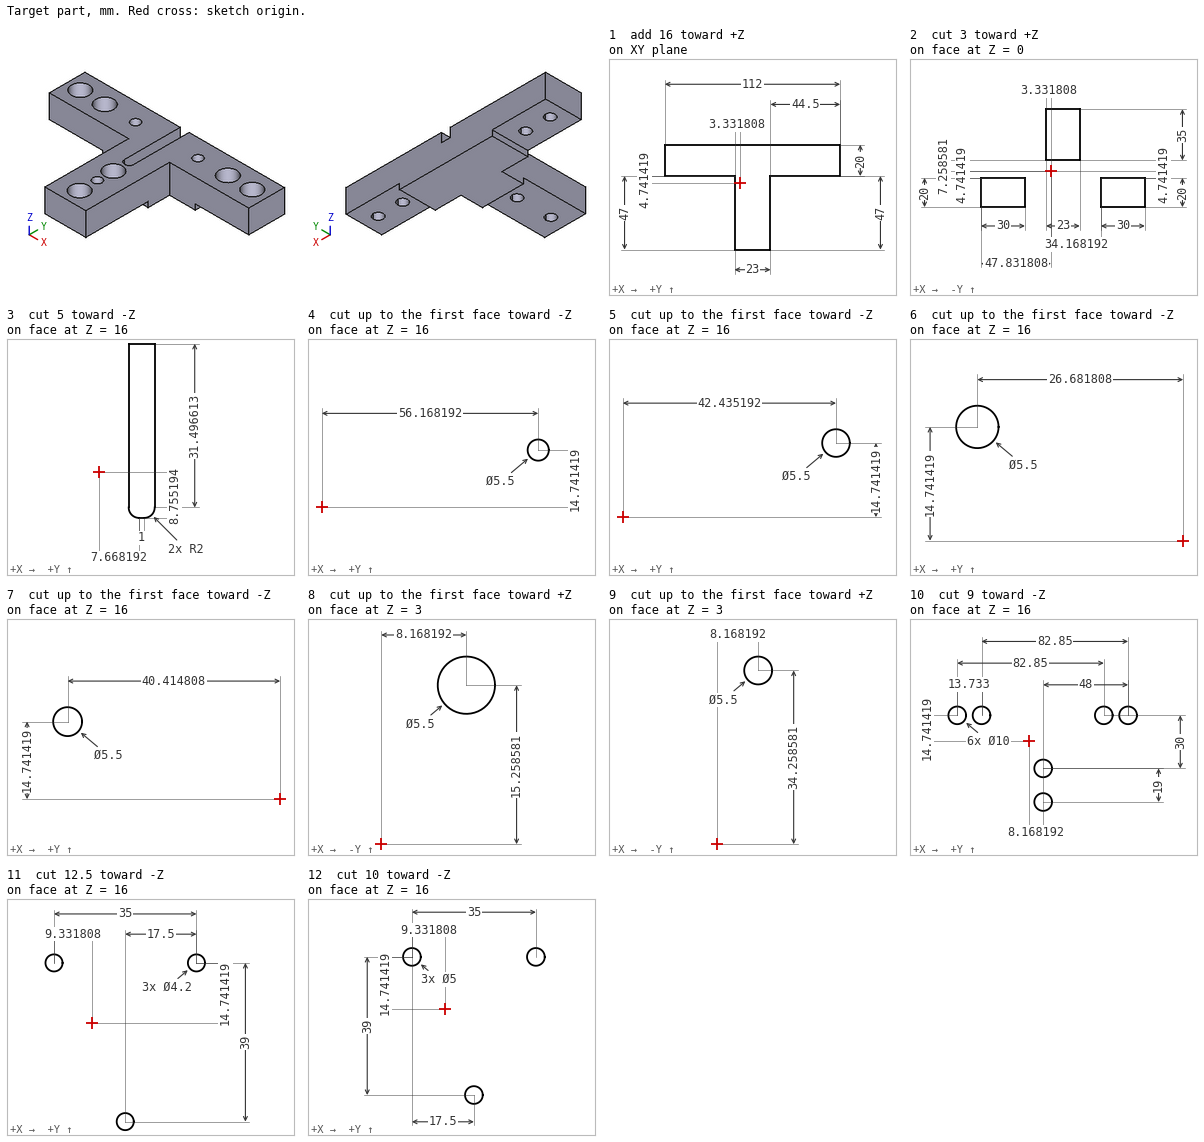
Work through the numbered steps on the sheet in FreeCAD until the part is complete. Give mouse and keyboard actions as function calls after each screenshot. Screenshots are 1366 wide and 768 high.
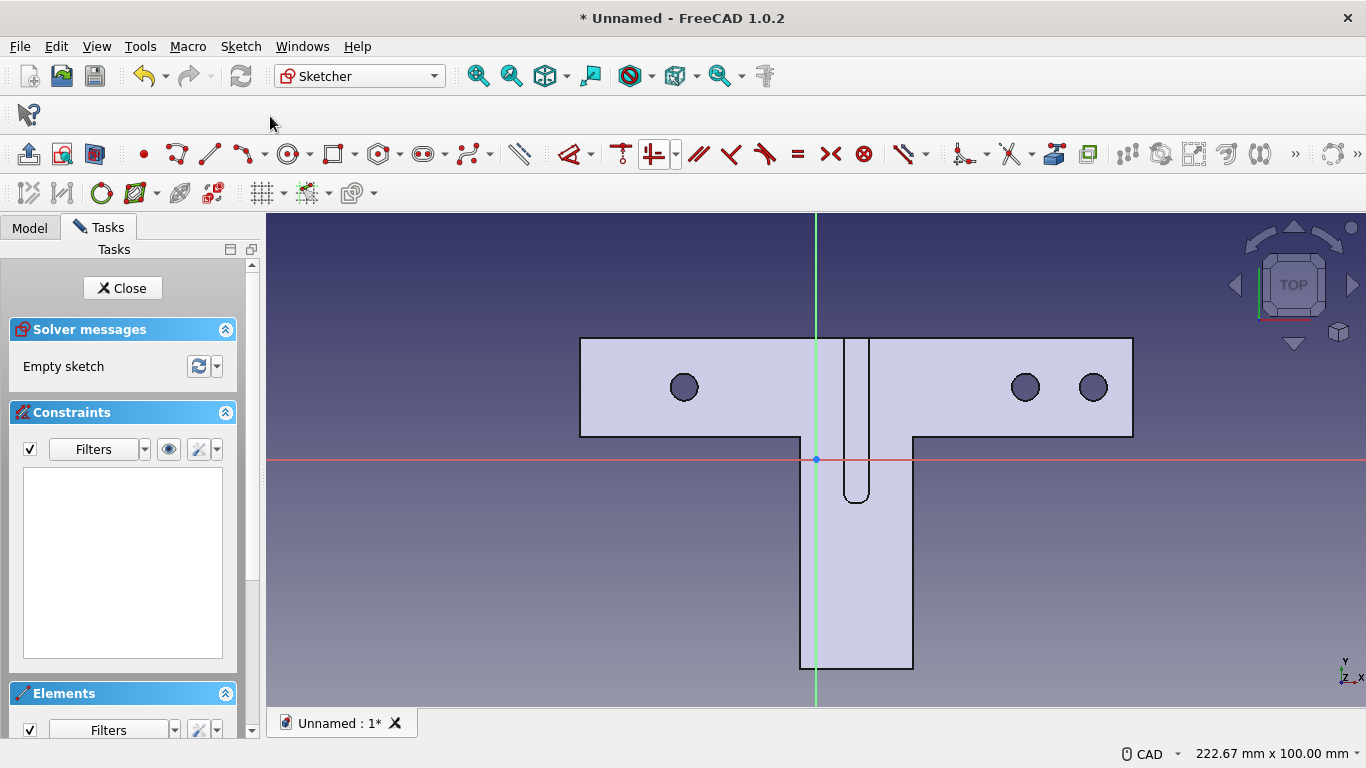
scroll(603, 380, up, 12)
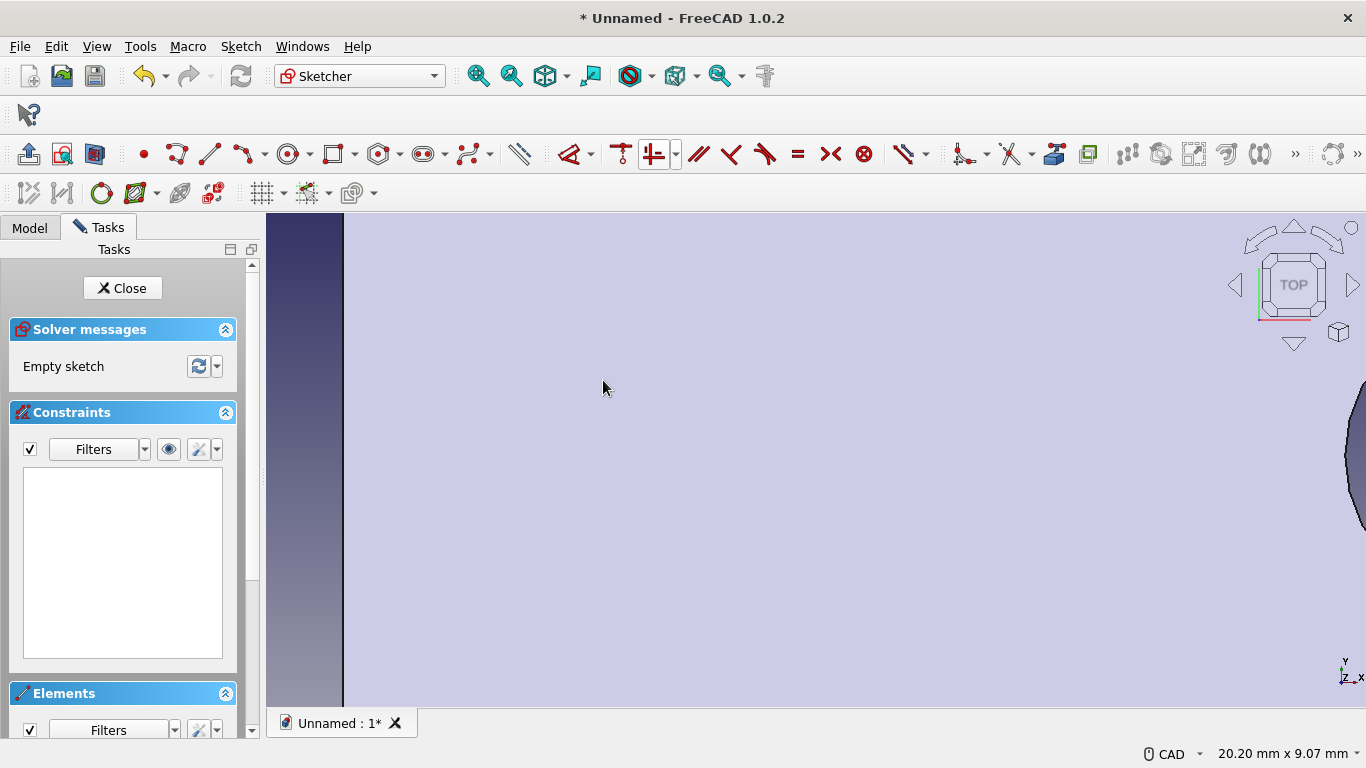
click(288, 154)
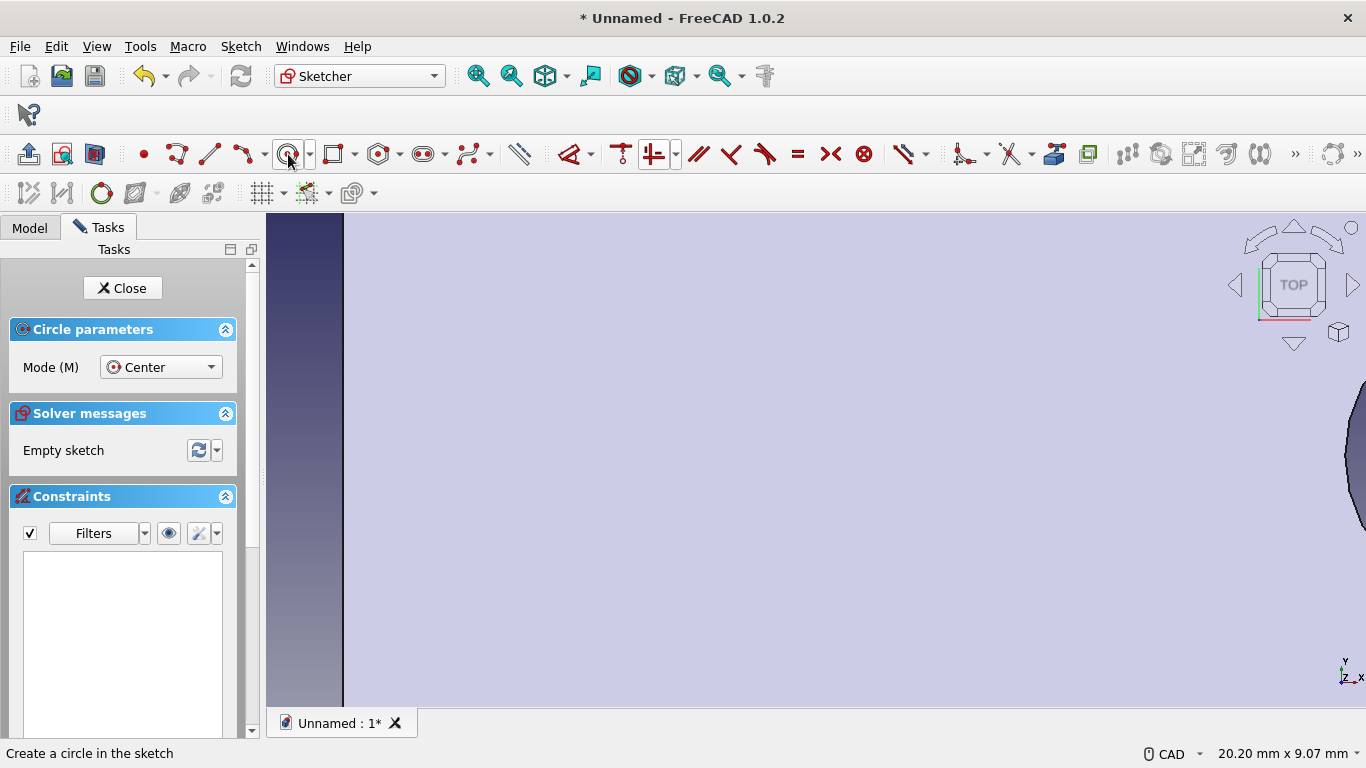
click(747, 456)
move(853, 350)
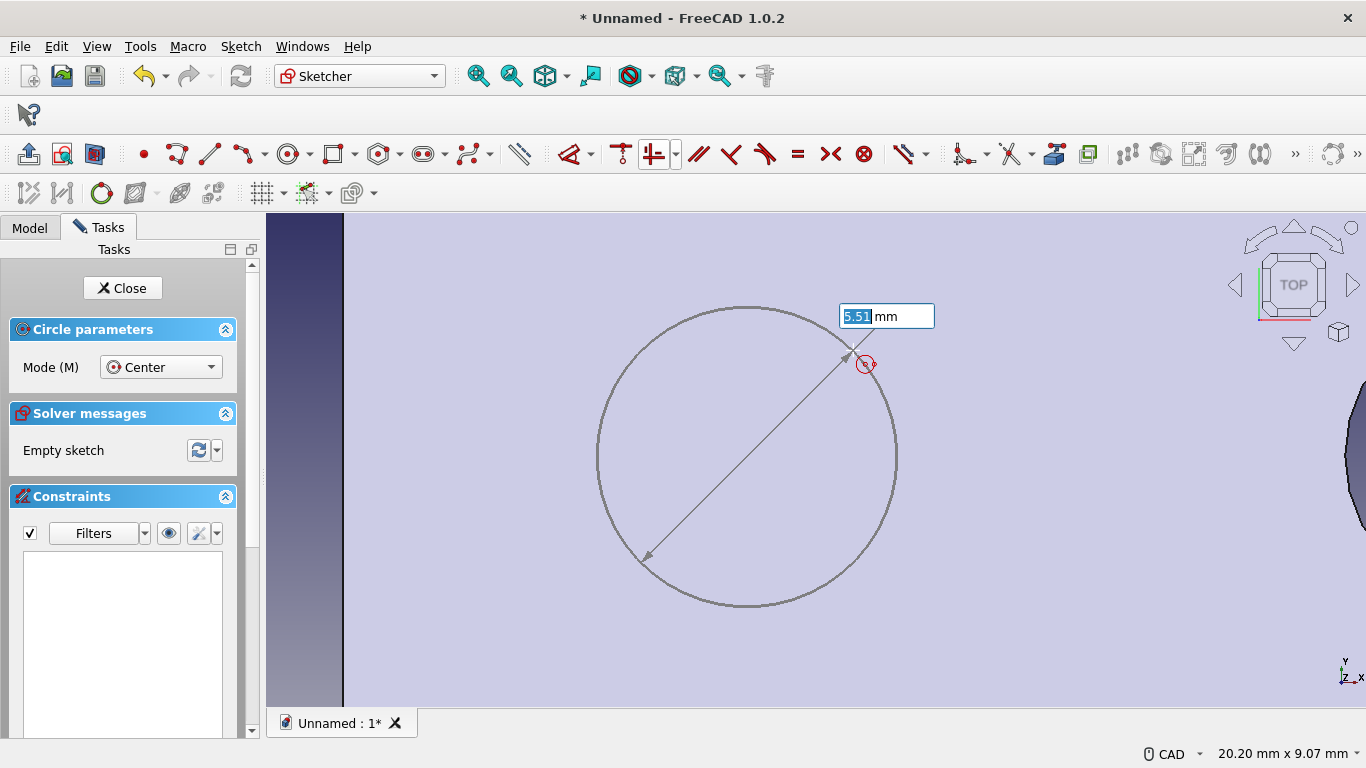
text(5.5)
key(Return)
key(Escape)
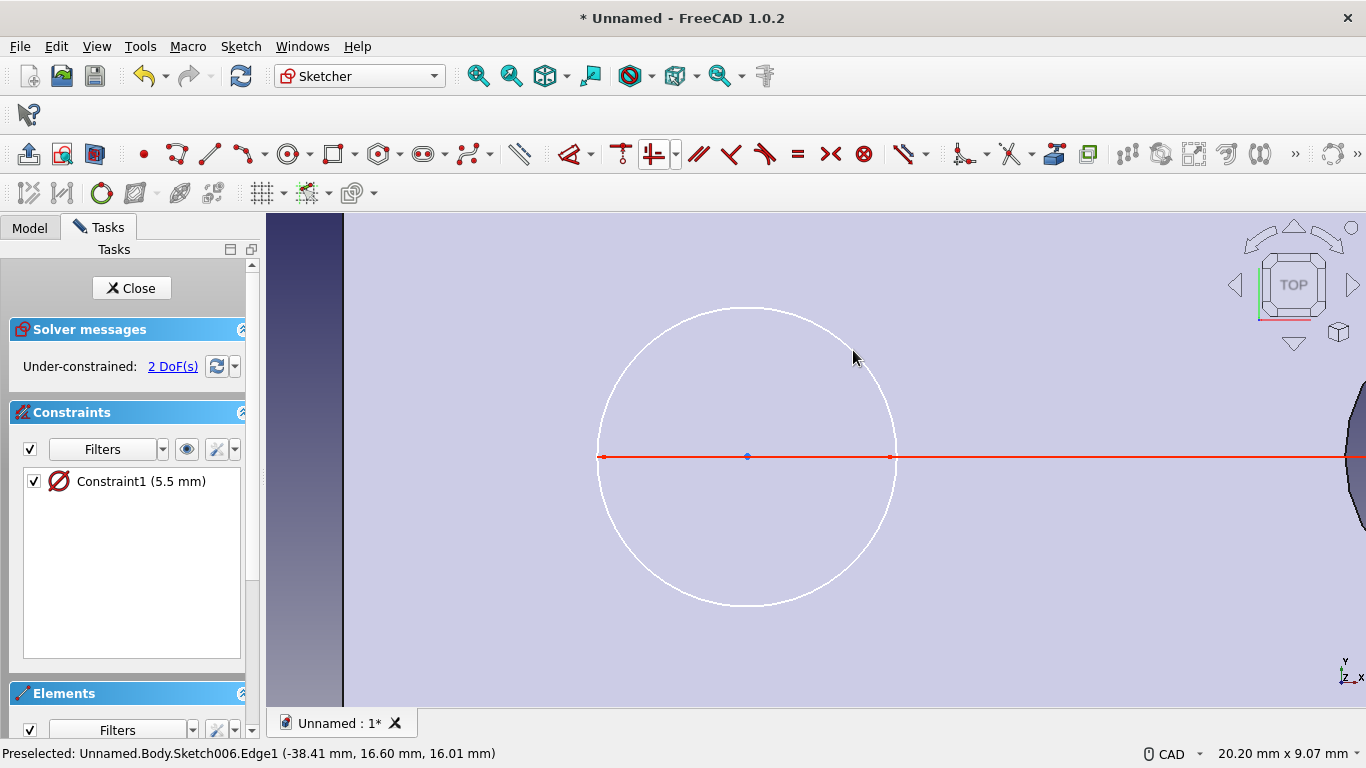
click(568, 154)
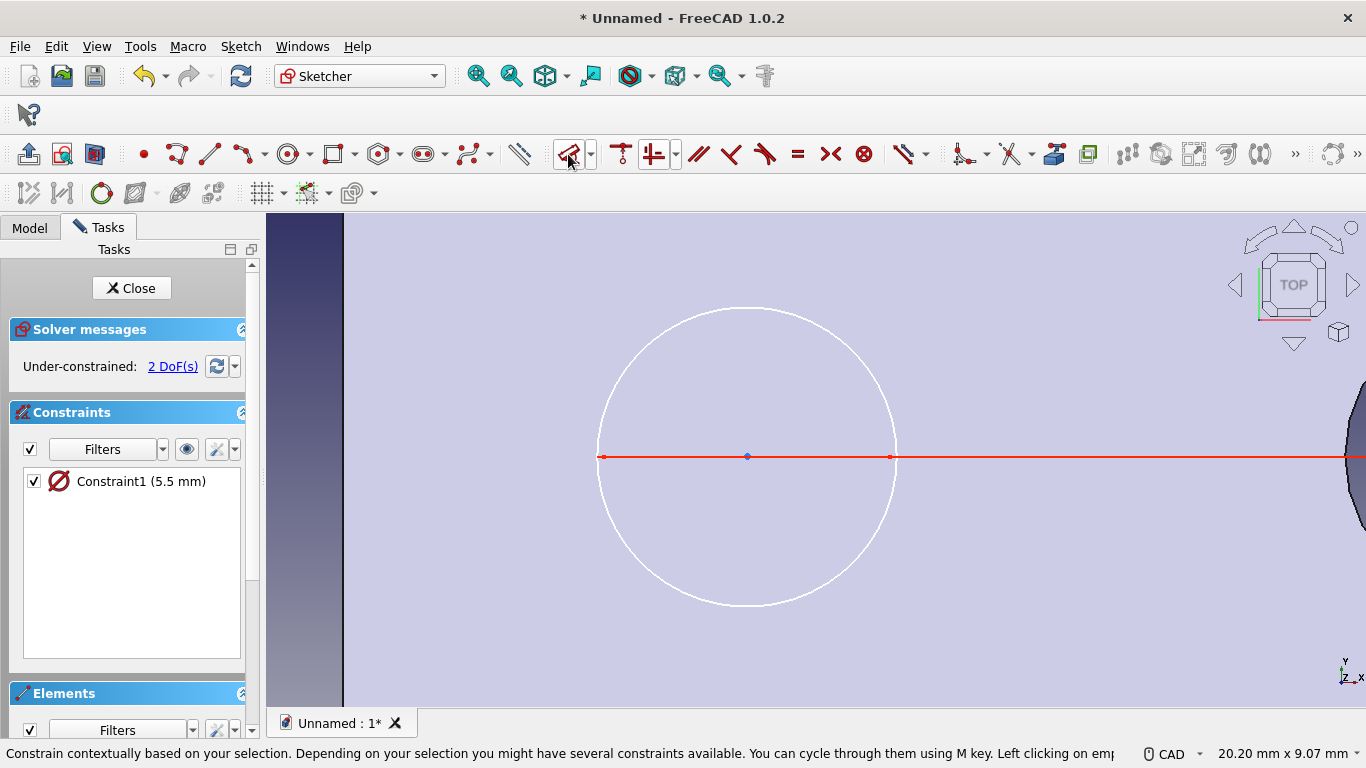
click(747, 457)
click(974, 423)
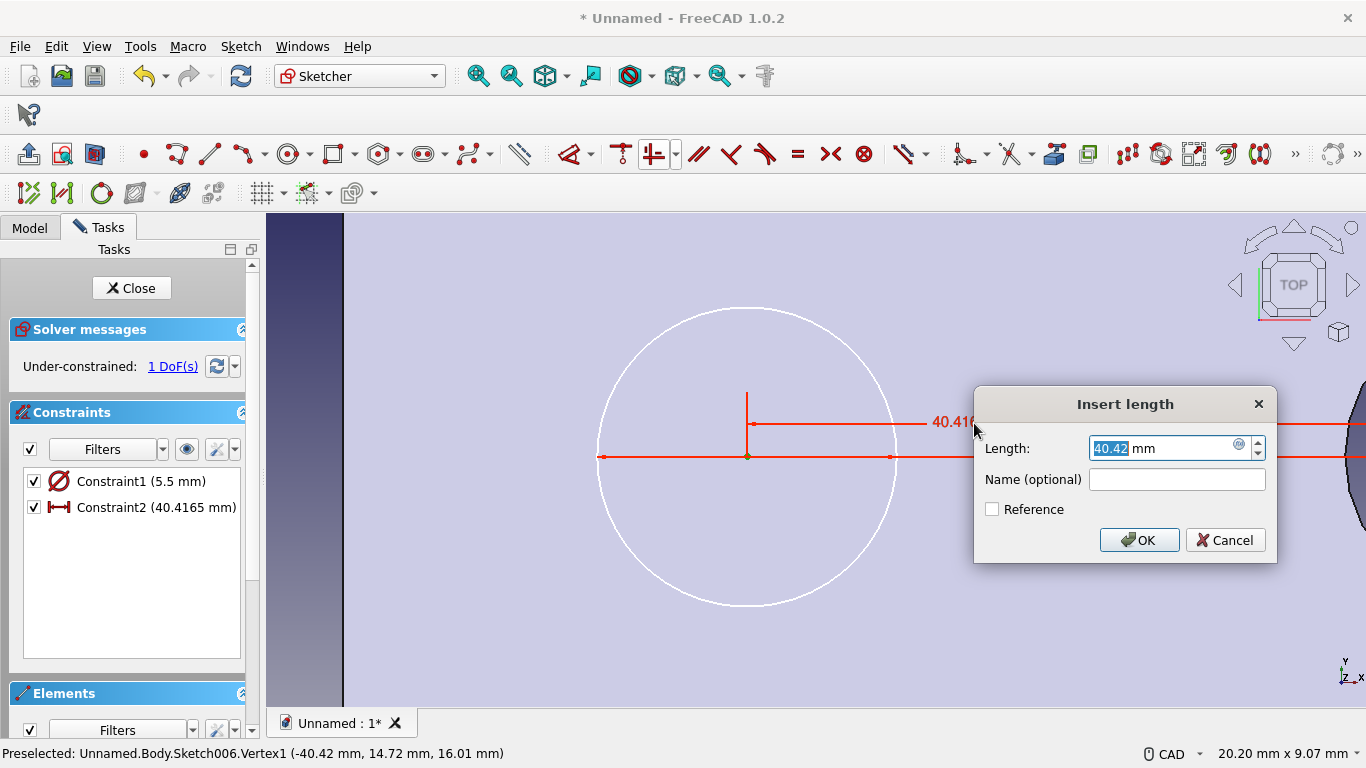
text(40.414808)
key(Return)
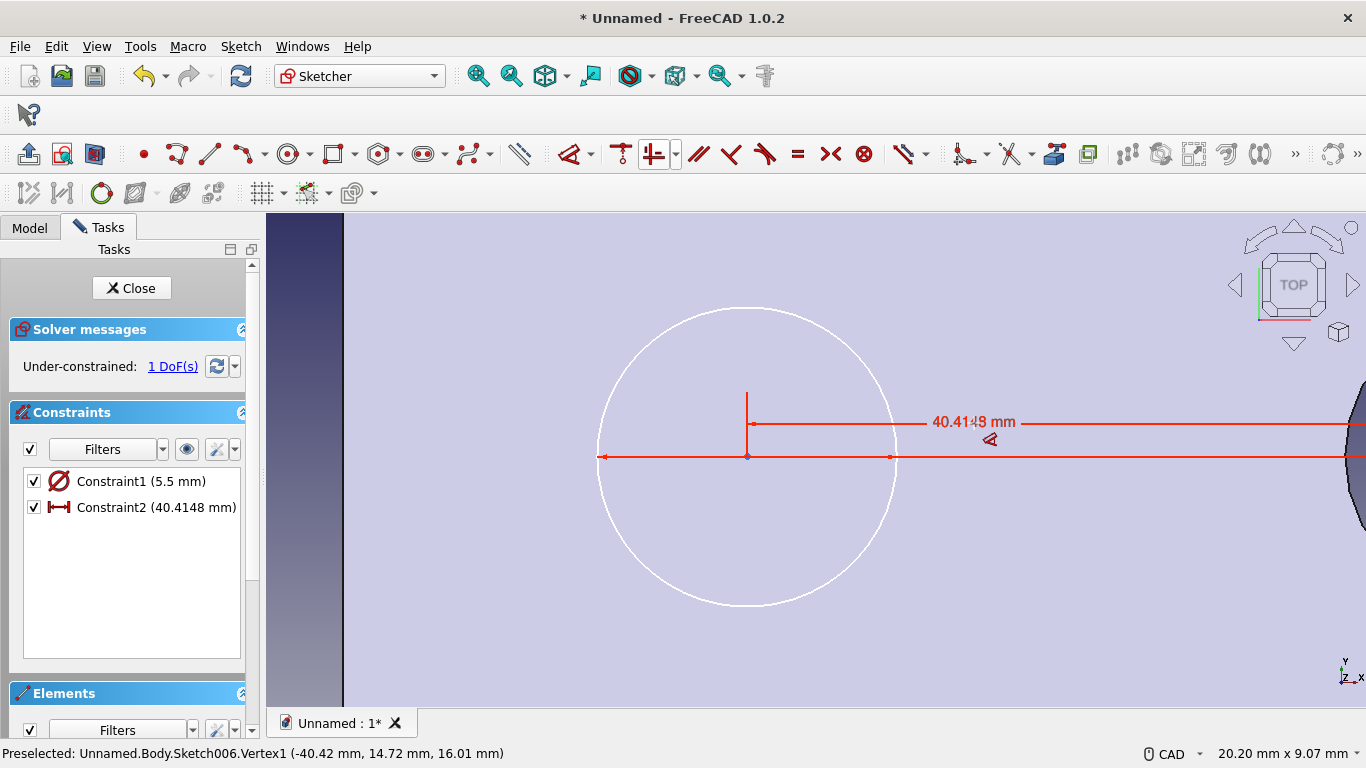
click(747, 457)
click(713, 568)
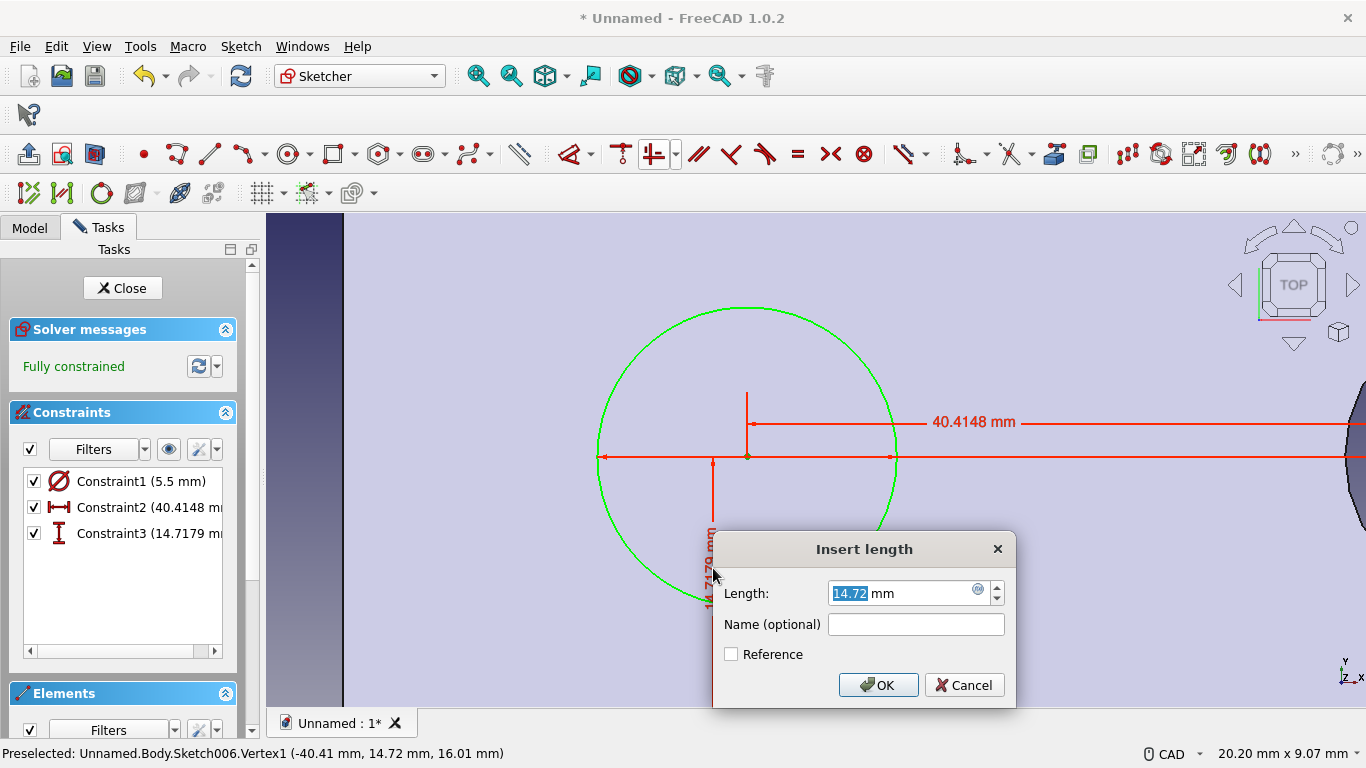
text(14.741419)
key(Return)
key(Escape)